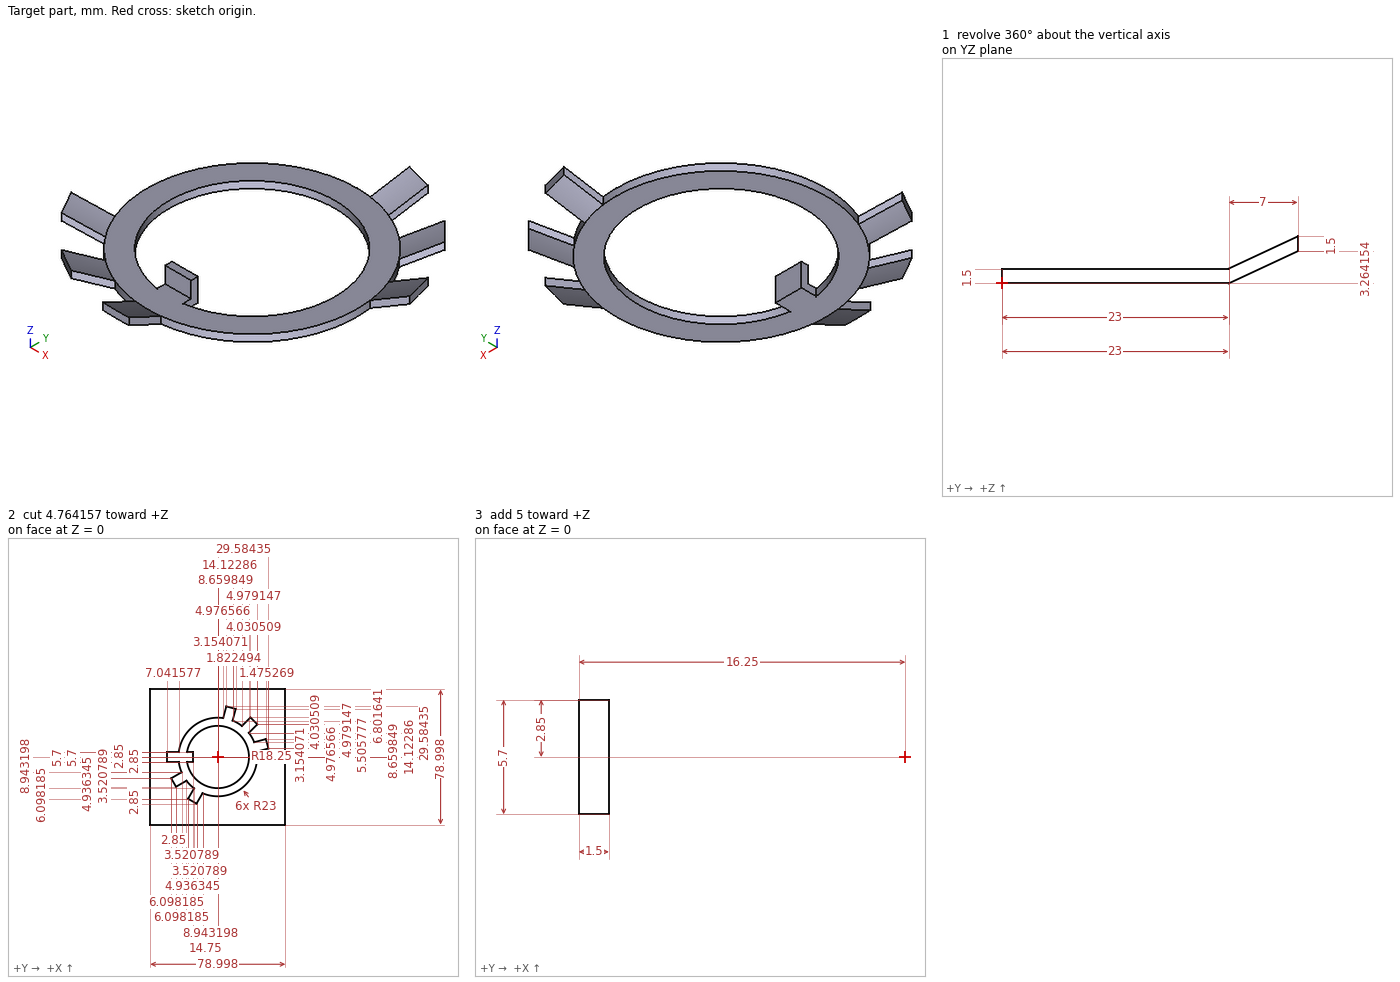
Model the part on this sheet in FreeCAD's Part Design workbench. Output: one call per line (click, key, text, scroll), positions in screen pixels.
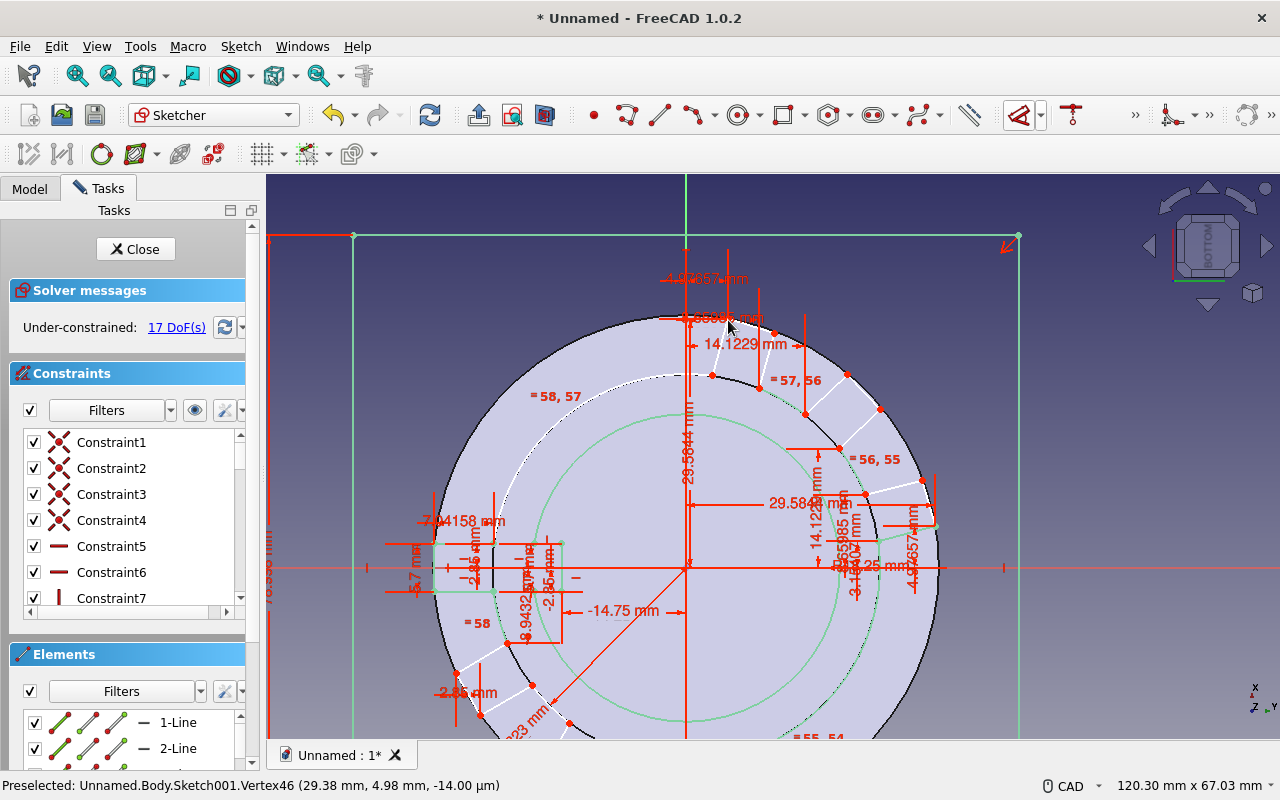
scroll(713, 376, up, 3)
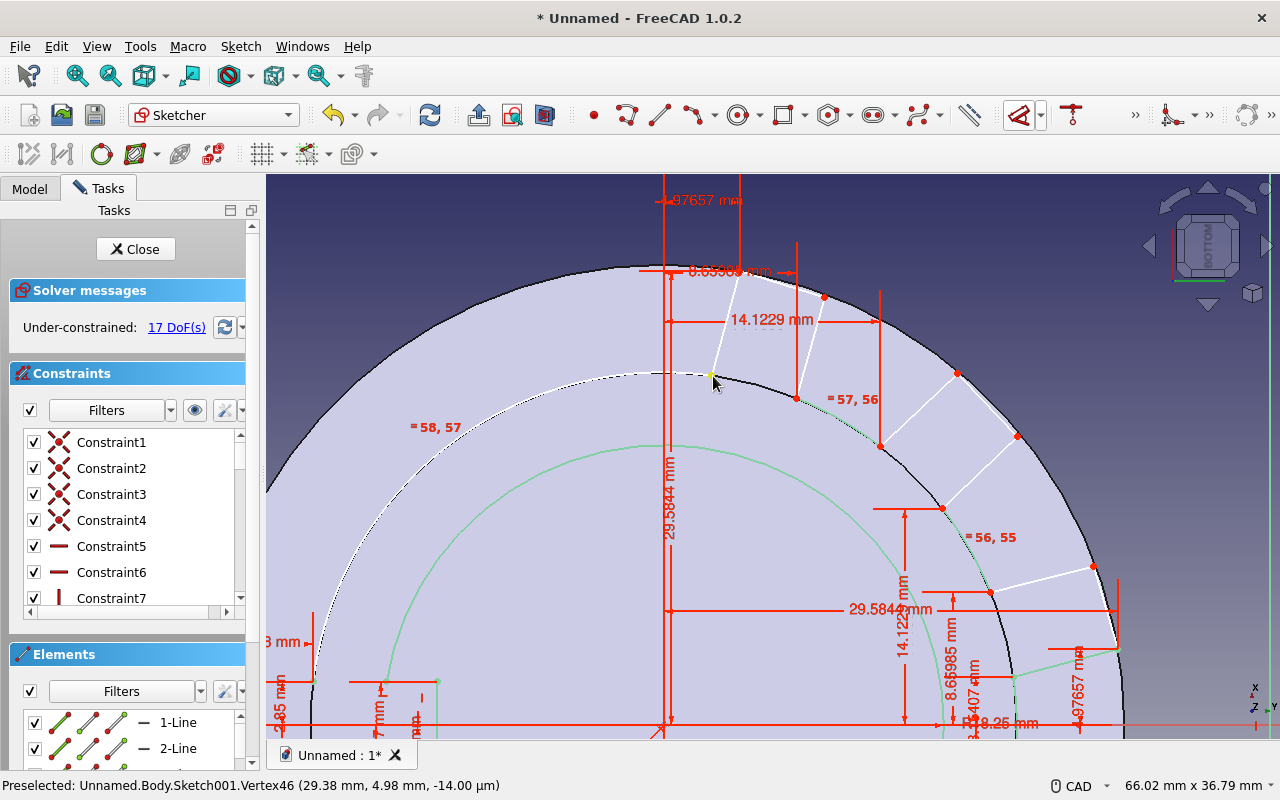
click(712, 376)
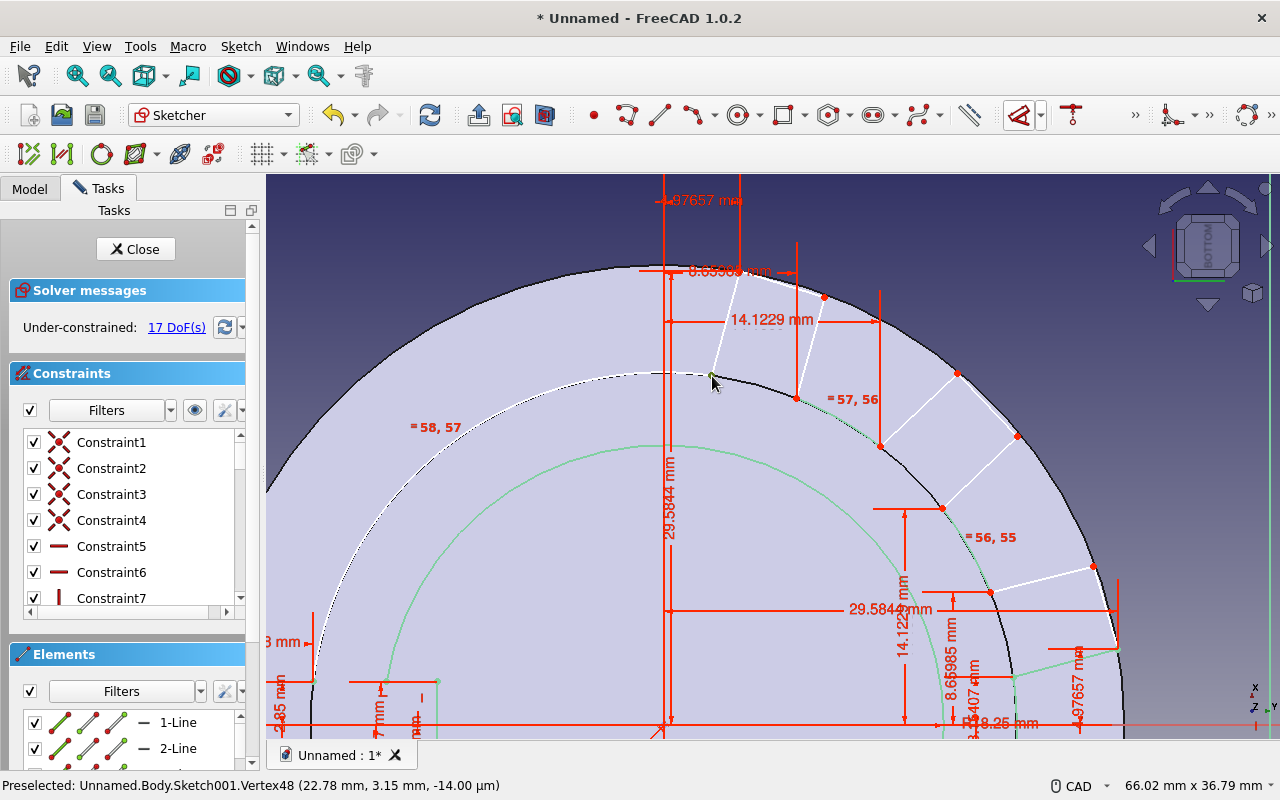
key(l)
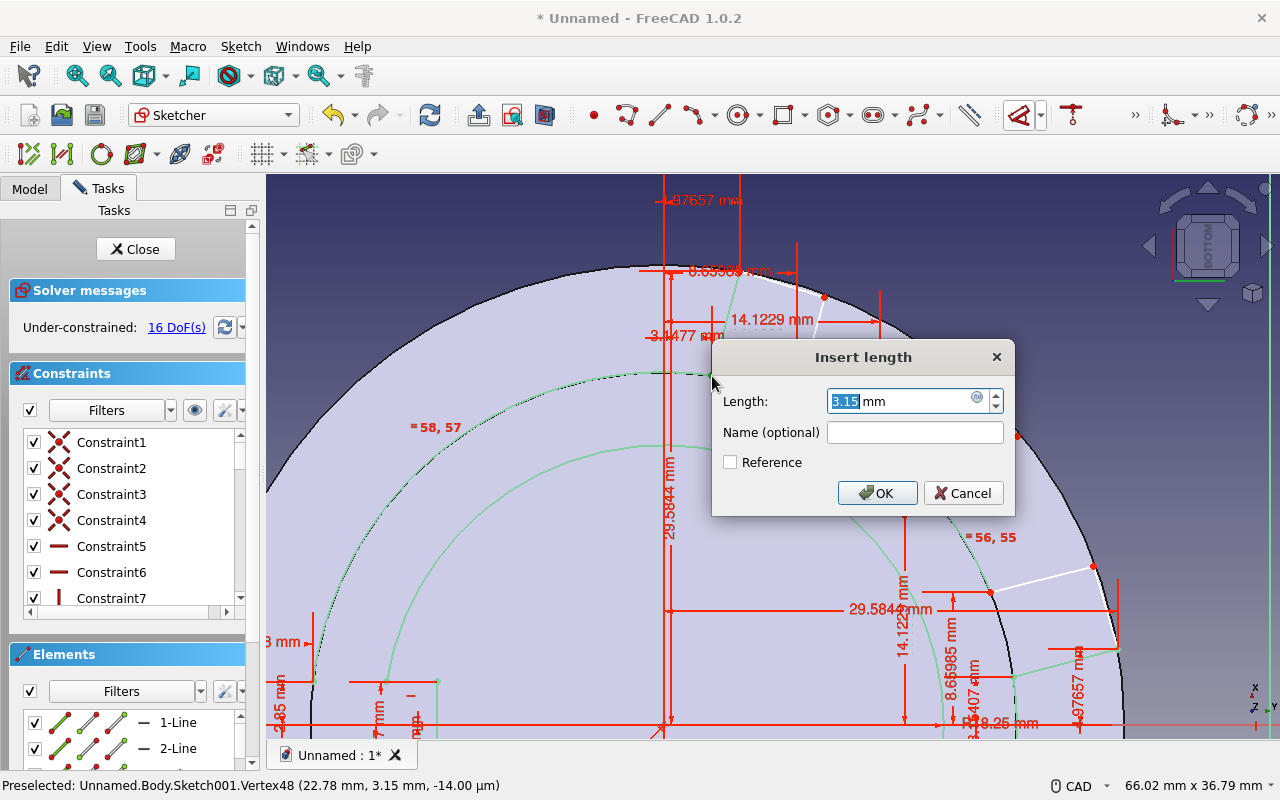
text(3.154071)
key(Return)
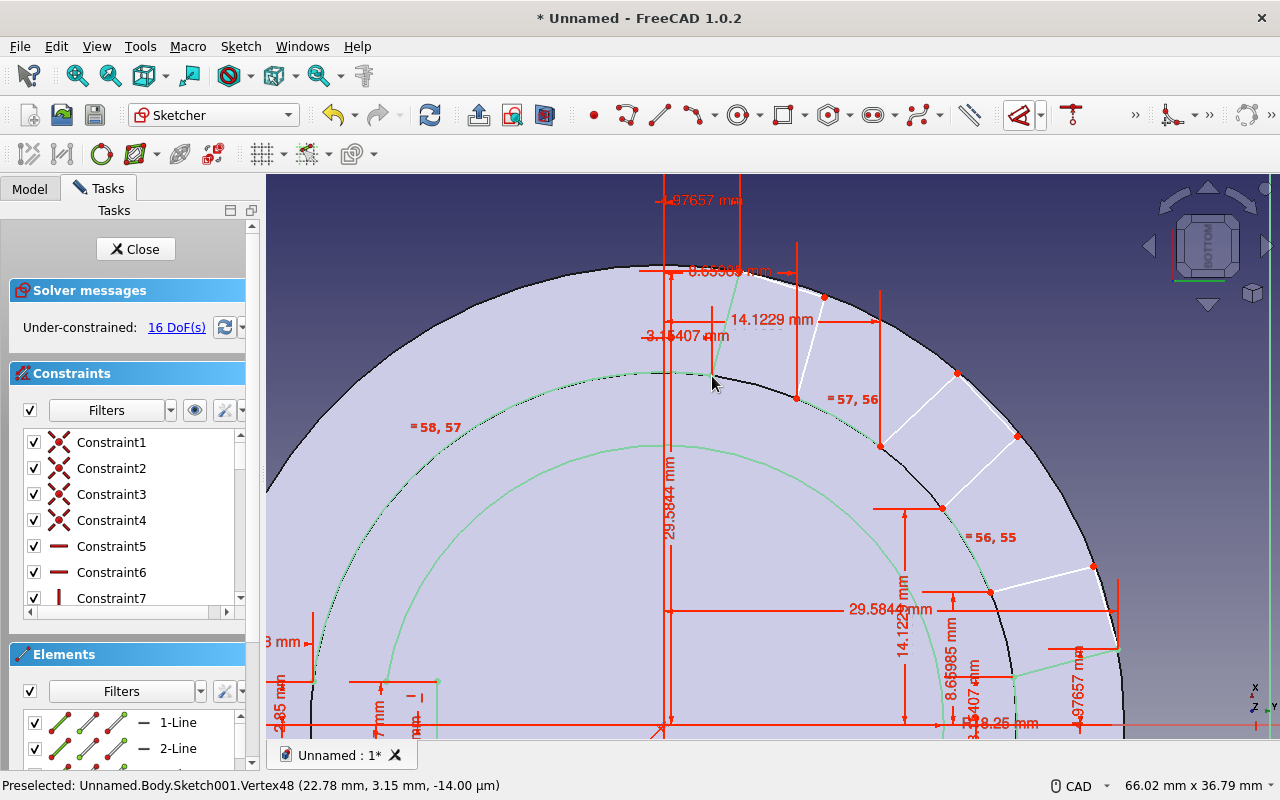
scroll(722, 341, down, 6)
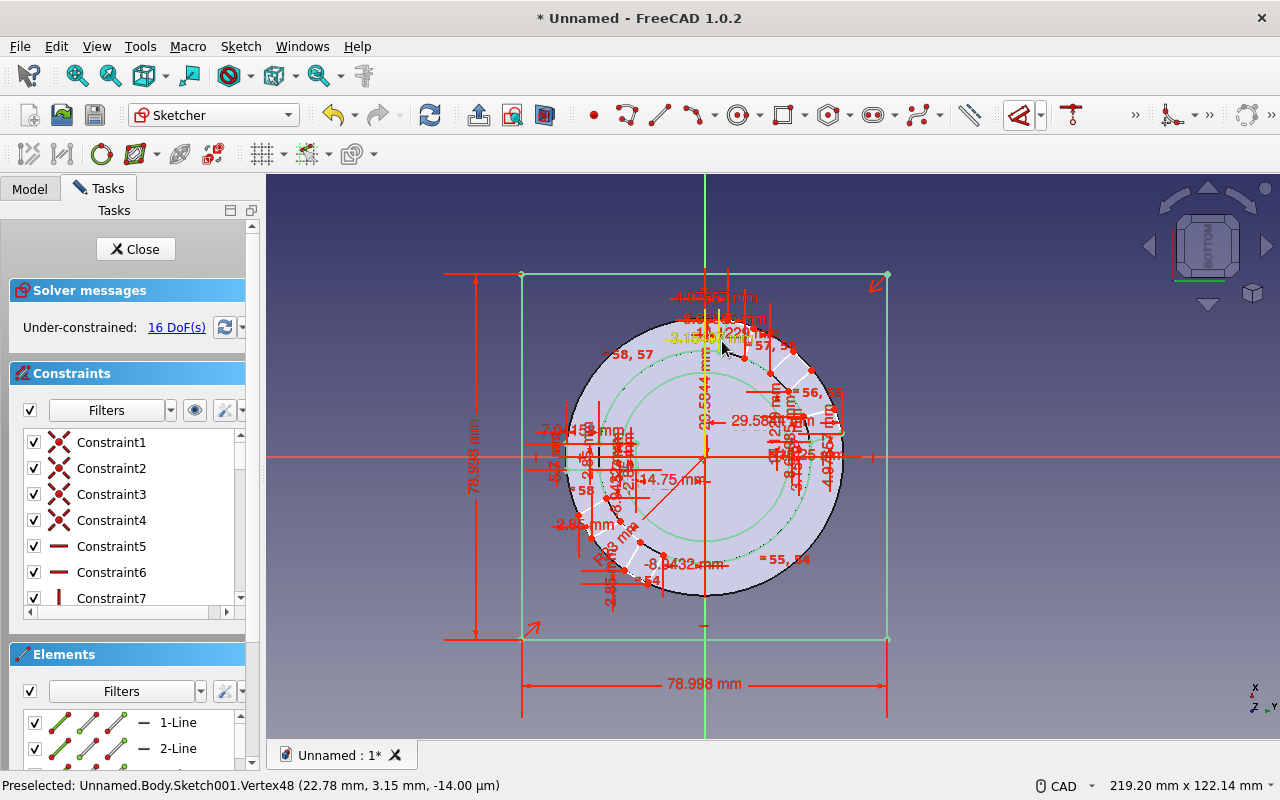
scroll(598, 503, up, 2)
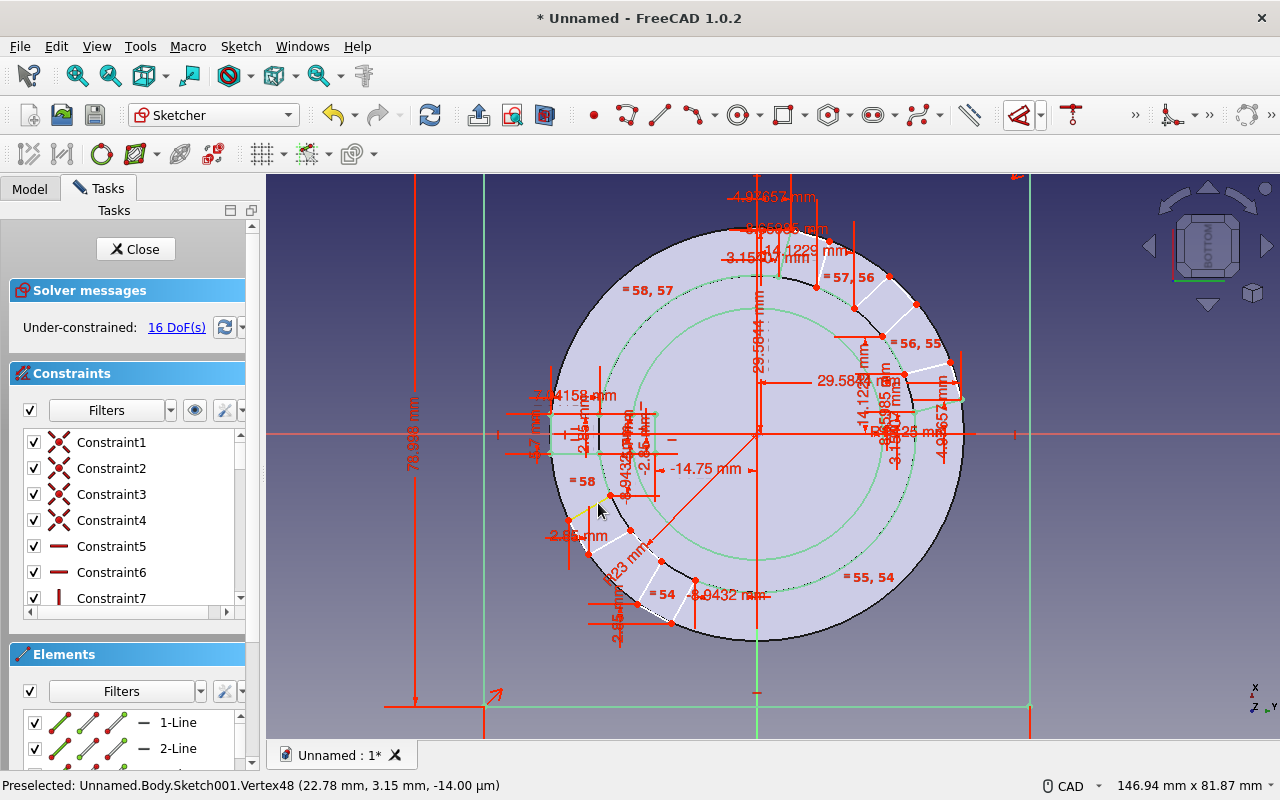
click(598, 503)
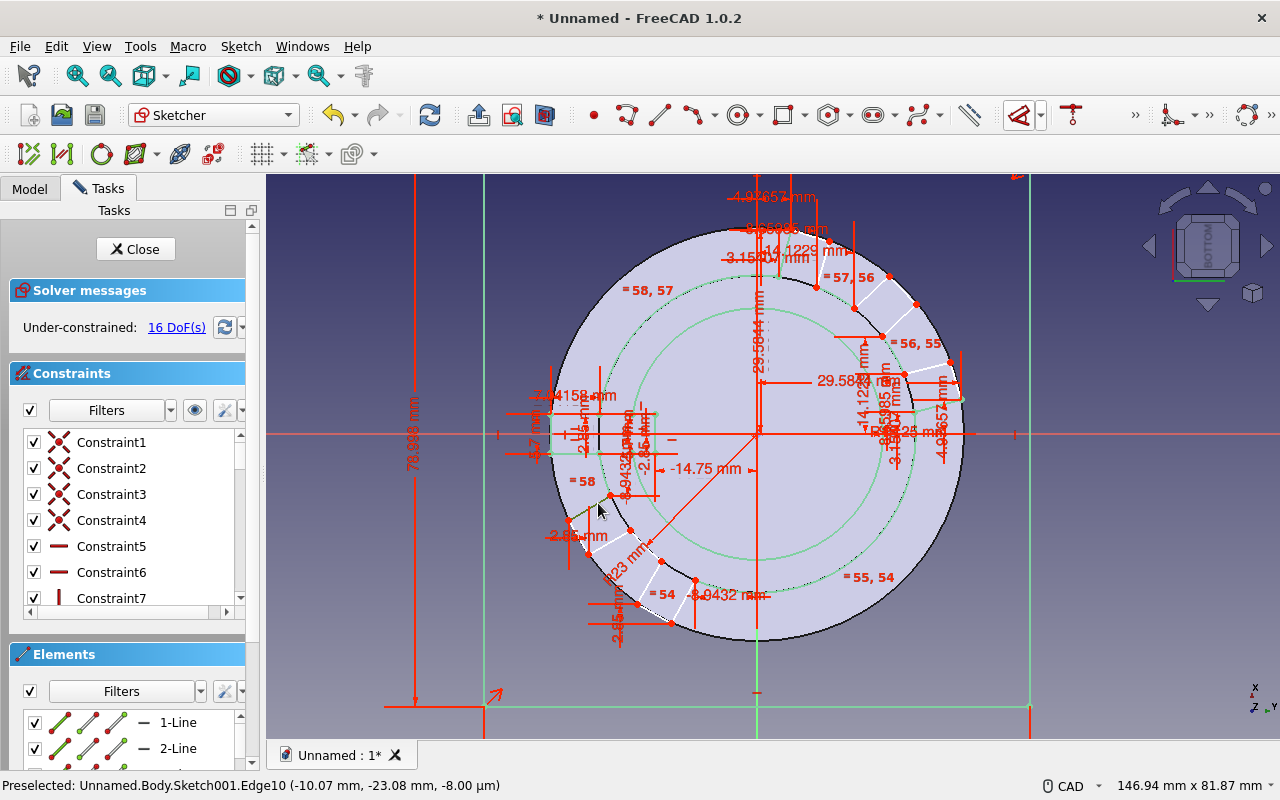
key(l)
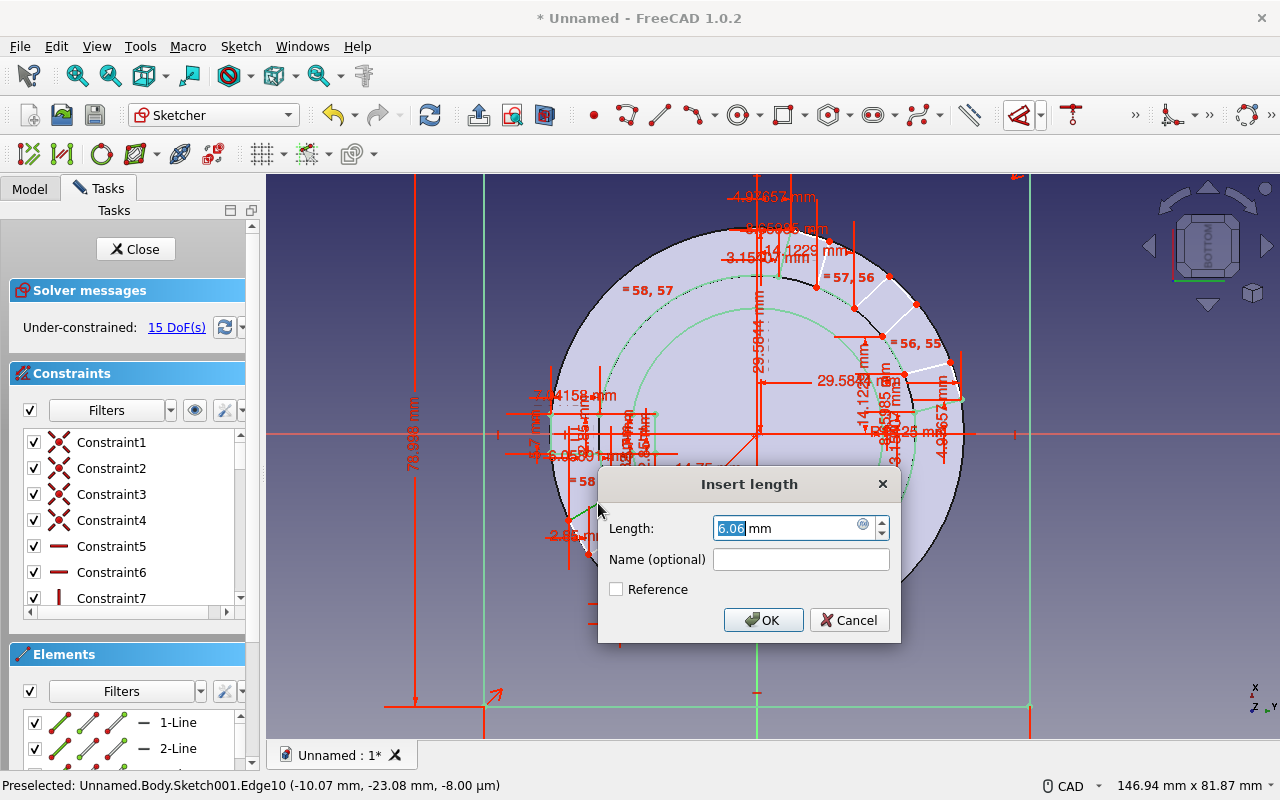
text(6.098185)
key(Return)